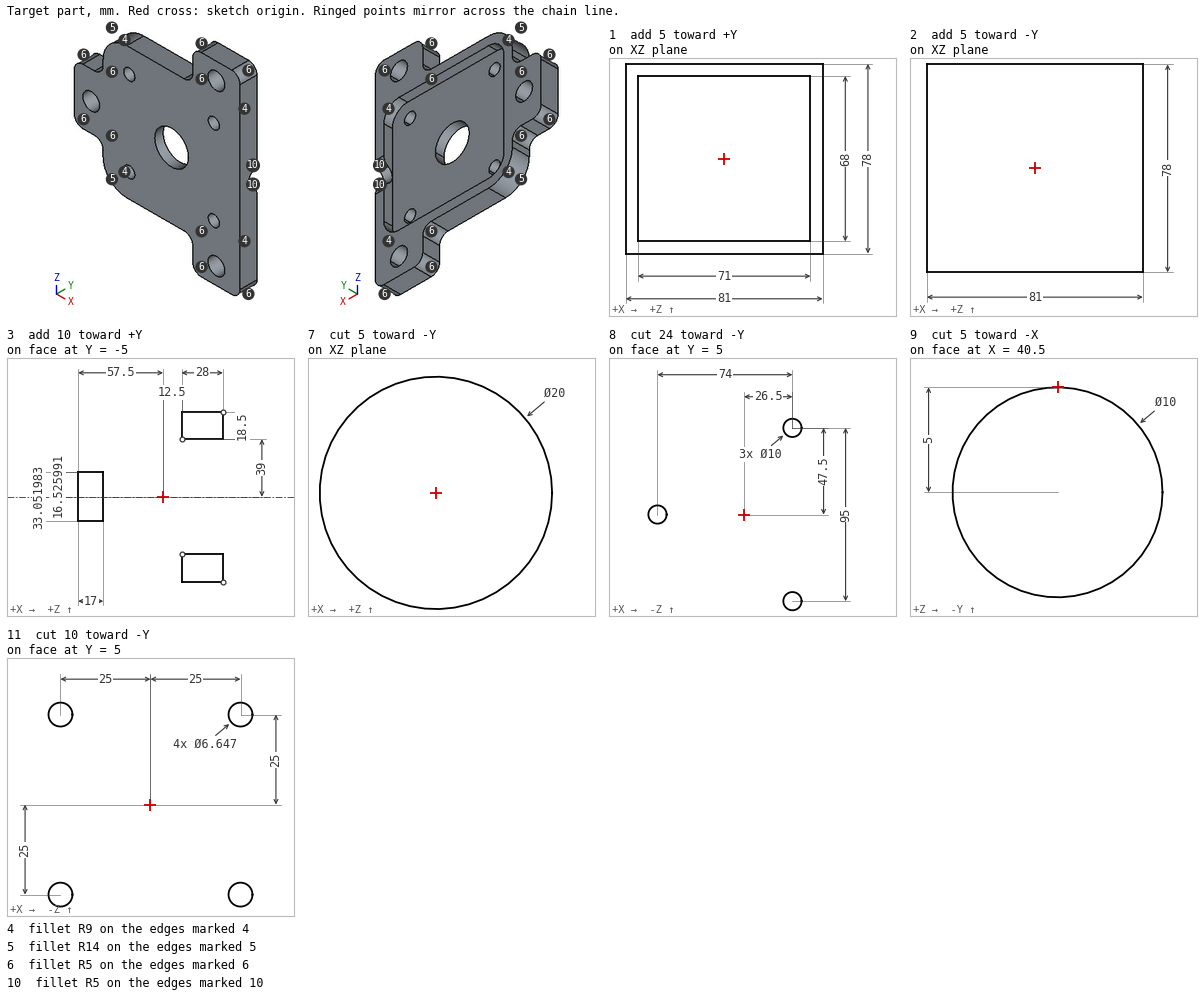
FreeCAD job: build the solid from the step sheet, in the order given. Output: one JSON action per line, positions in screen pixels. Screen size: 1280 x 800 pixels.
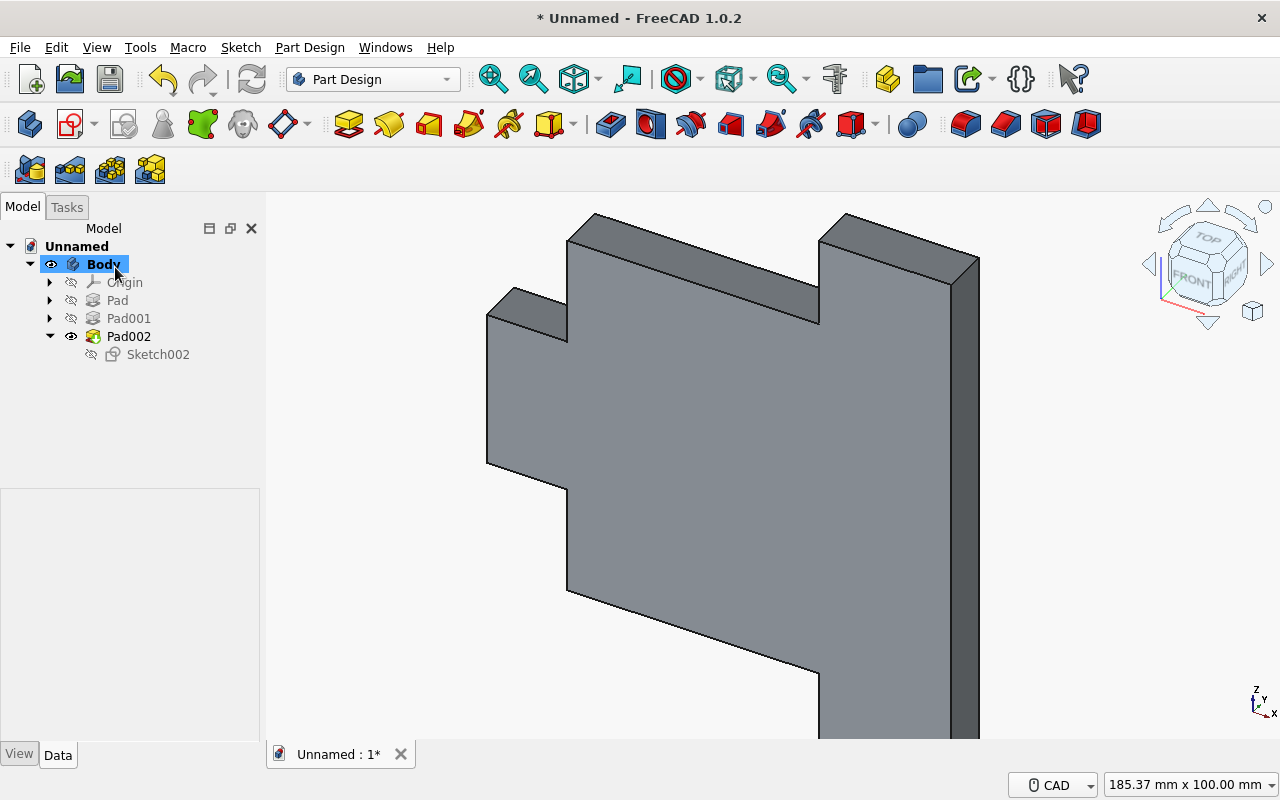
{"action": "key", "text": "v f"}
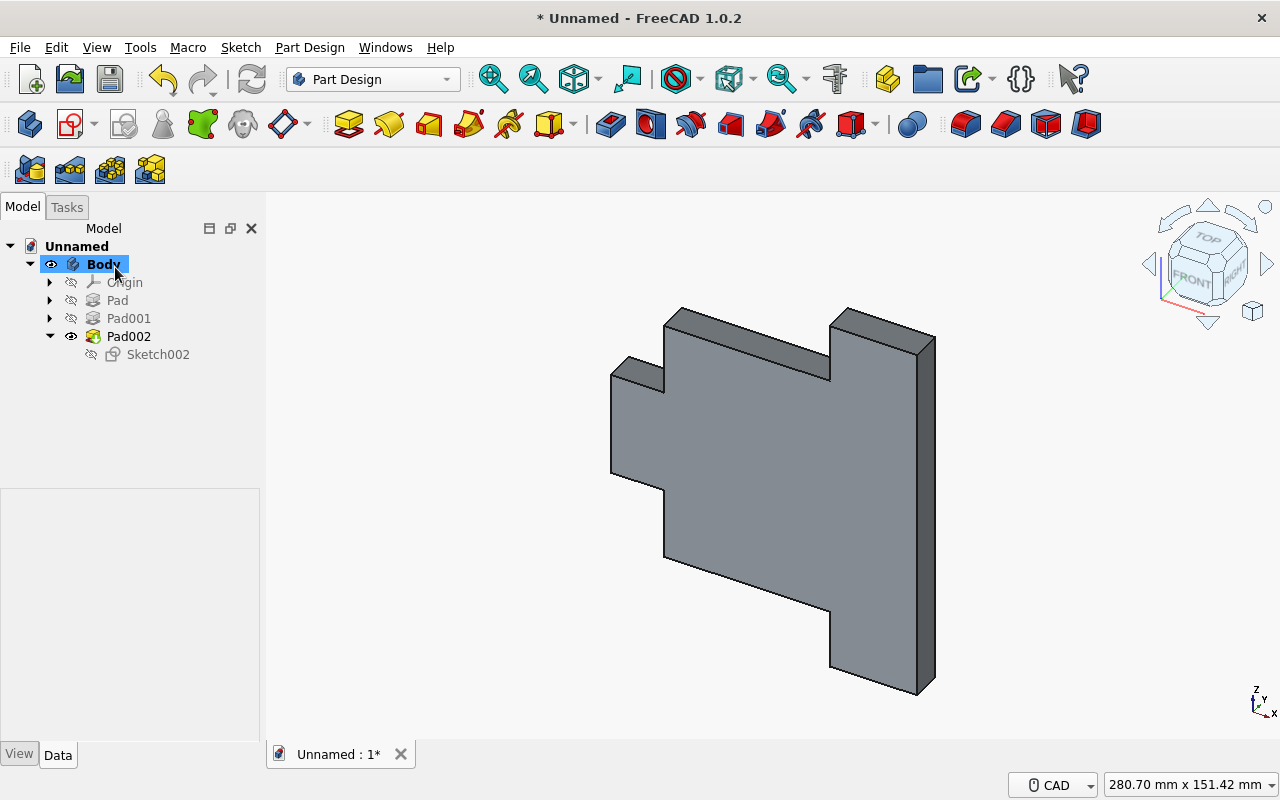
{"action": "scroll", "coordinate": [915, 405], "scroll_direction": "up", "scroll_amount": 4}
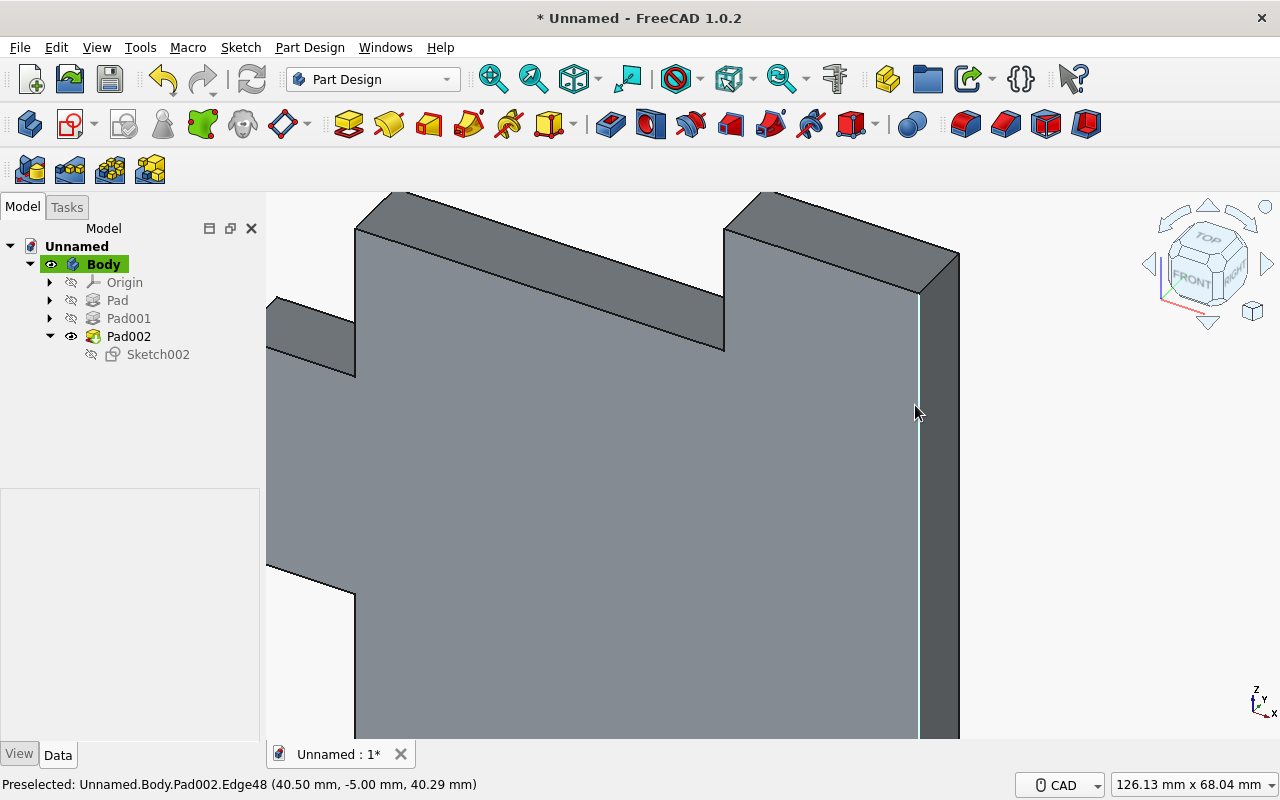
{"action": "key", "text": "v f"}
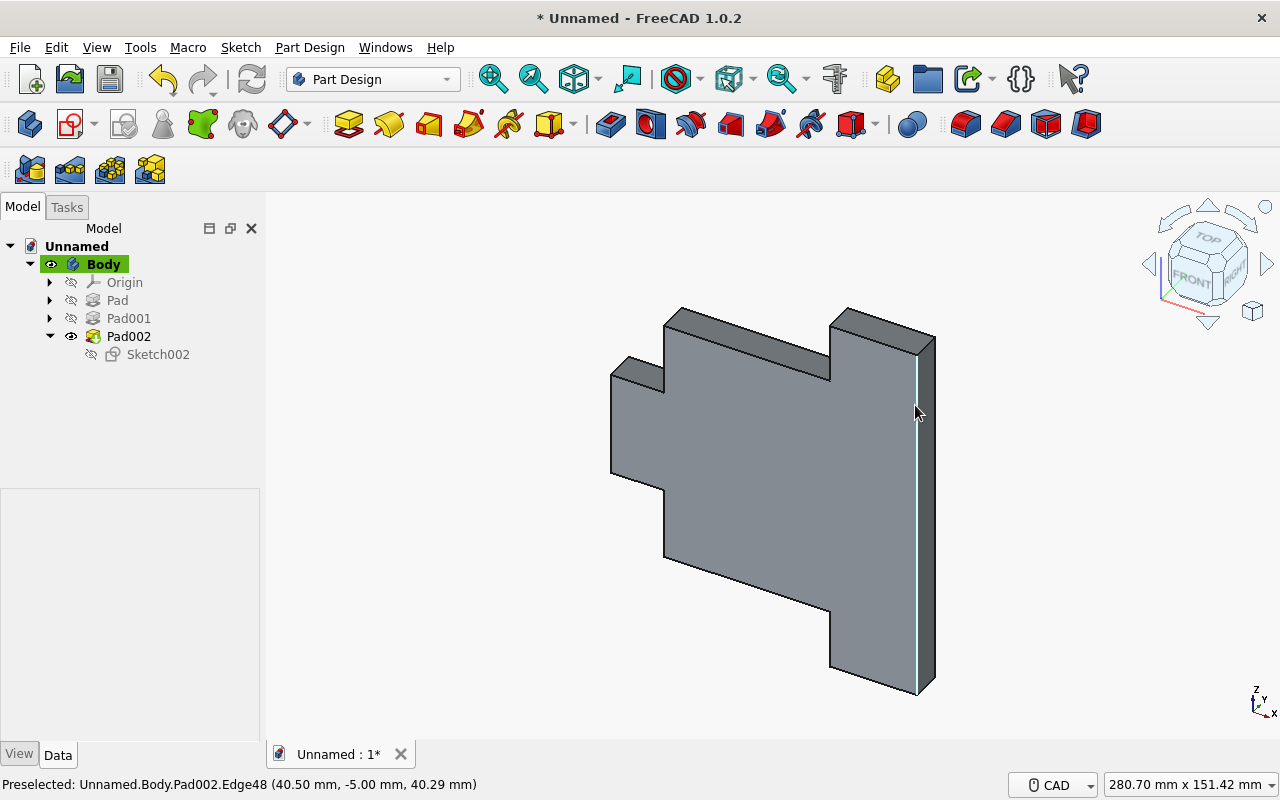
{"action": "key", "text": "0"}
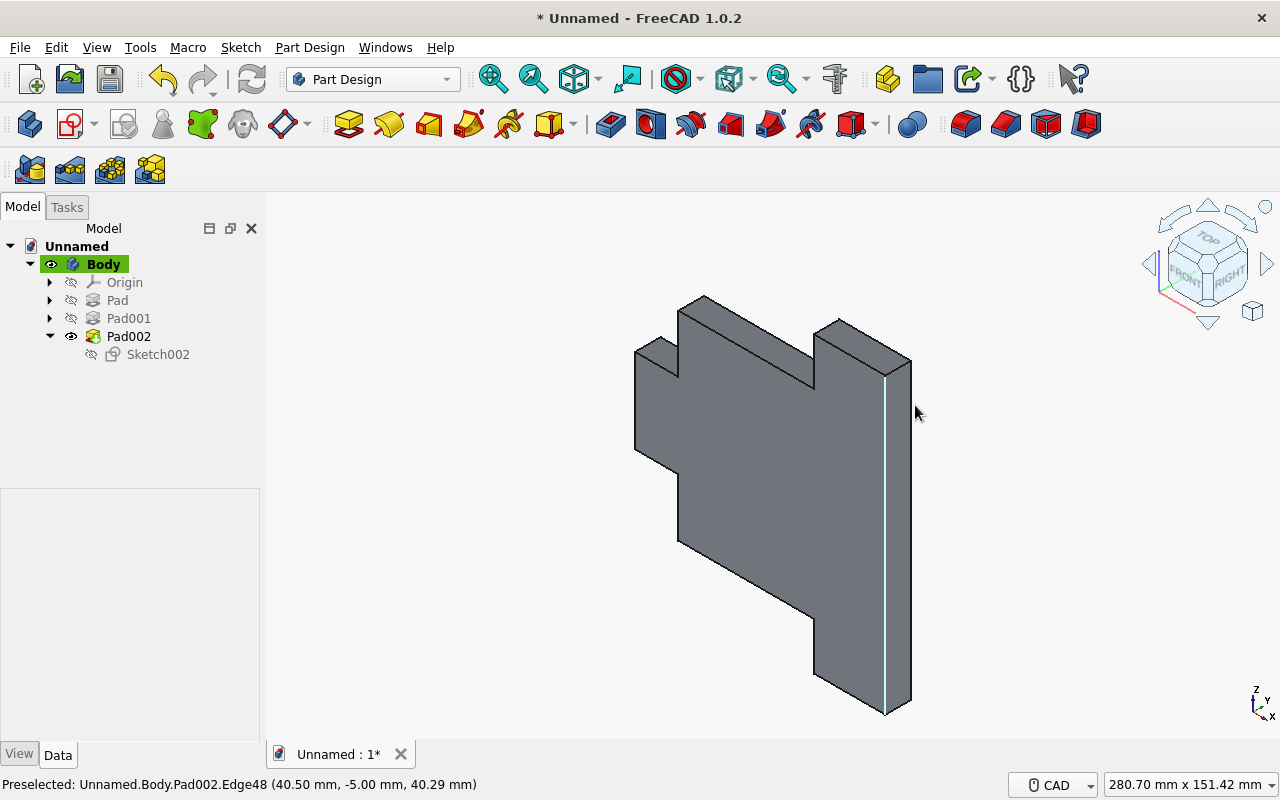
{"action": "scroll", "coordinate": [892, 425], "scroll_direction": "up", "scroll_amount": 4}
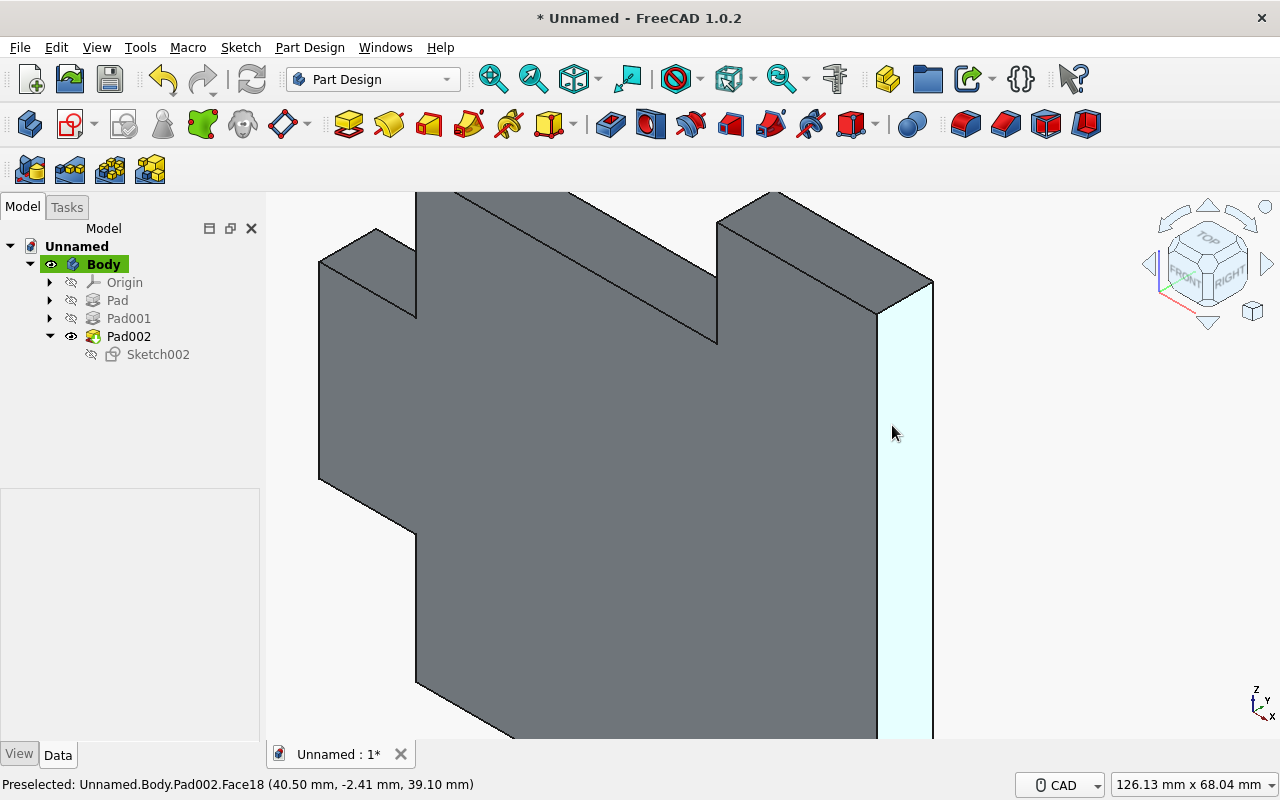
{"action": "key", "text": "v f"}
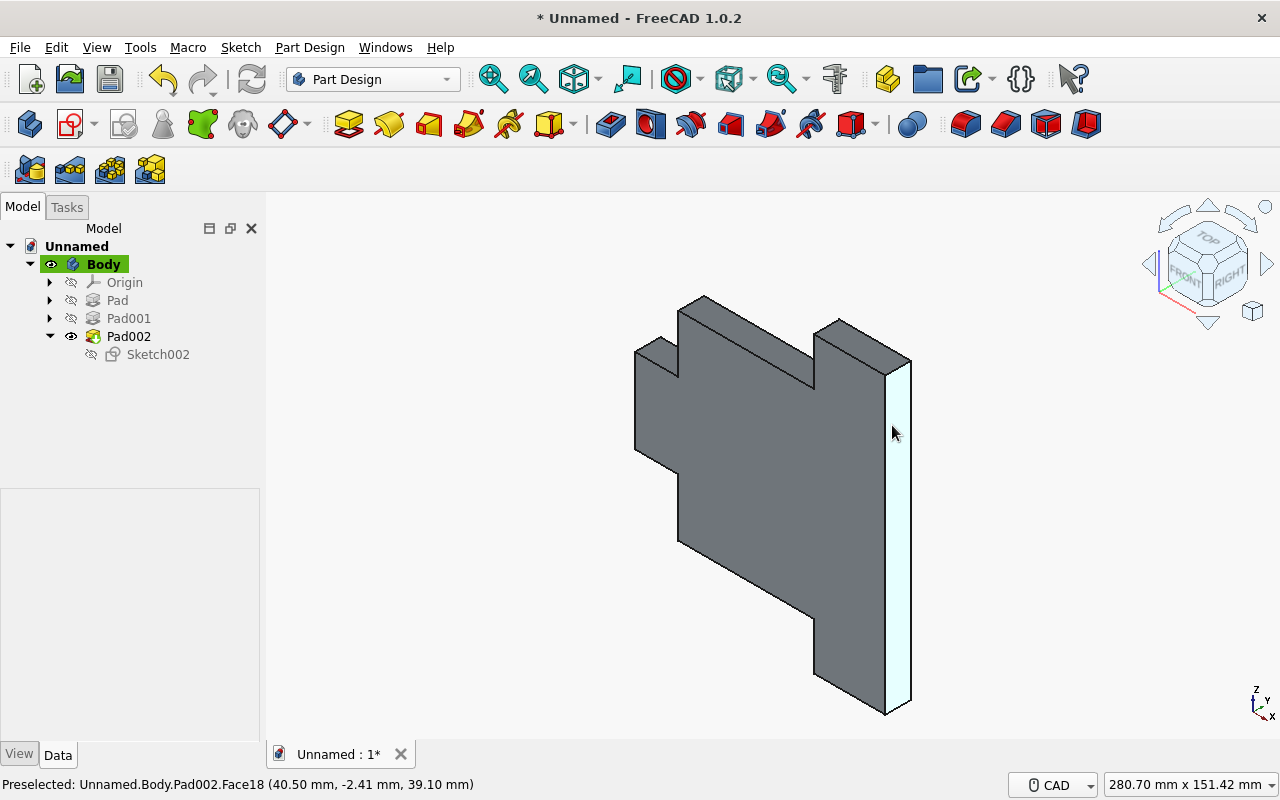
{"action": "key", "text": "2"}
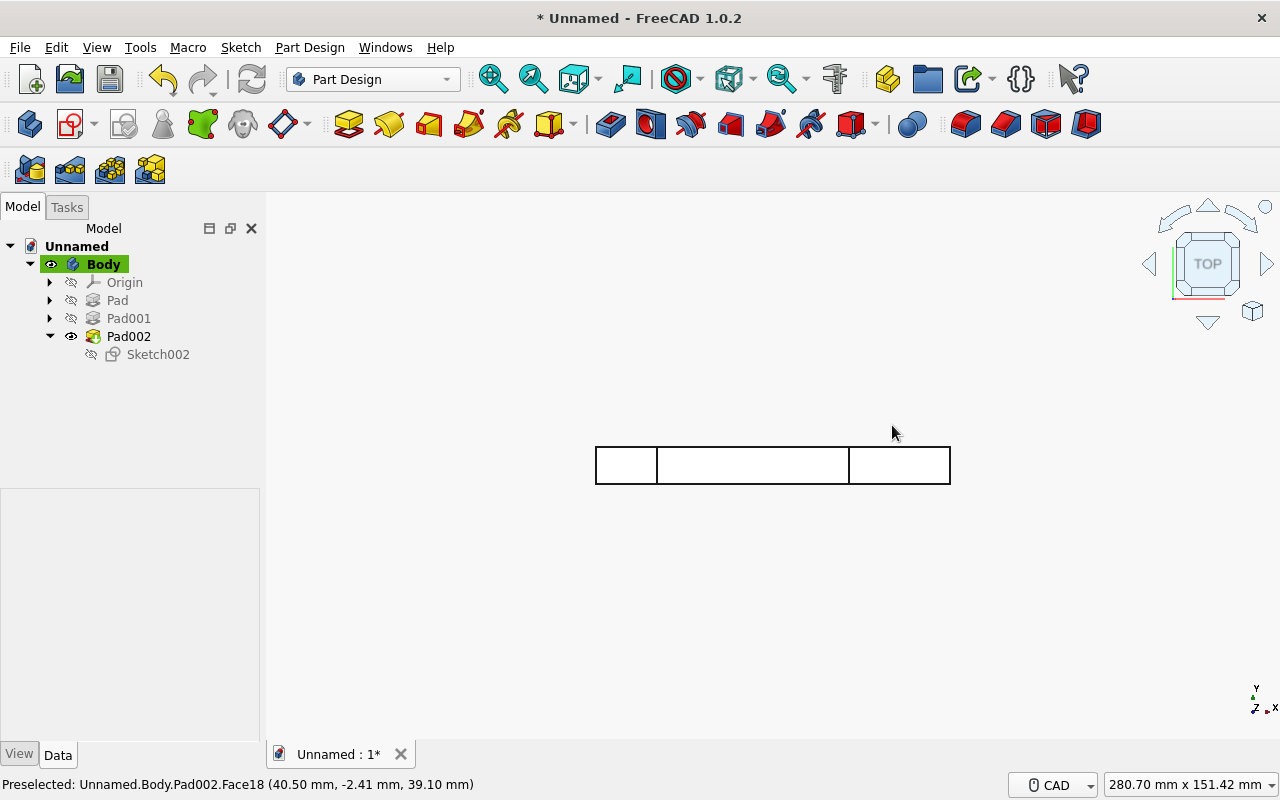
{"action": "left_click", "coordinate": [494, 80]}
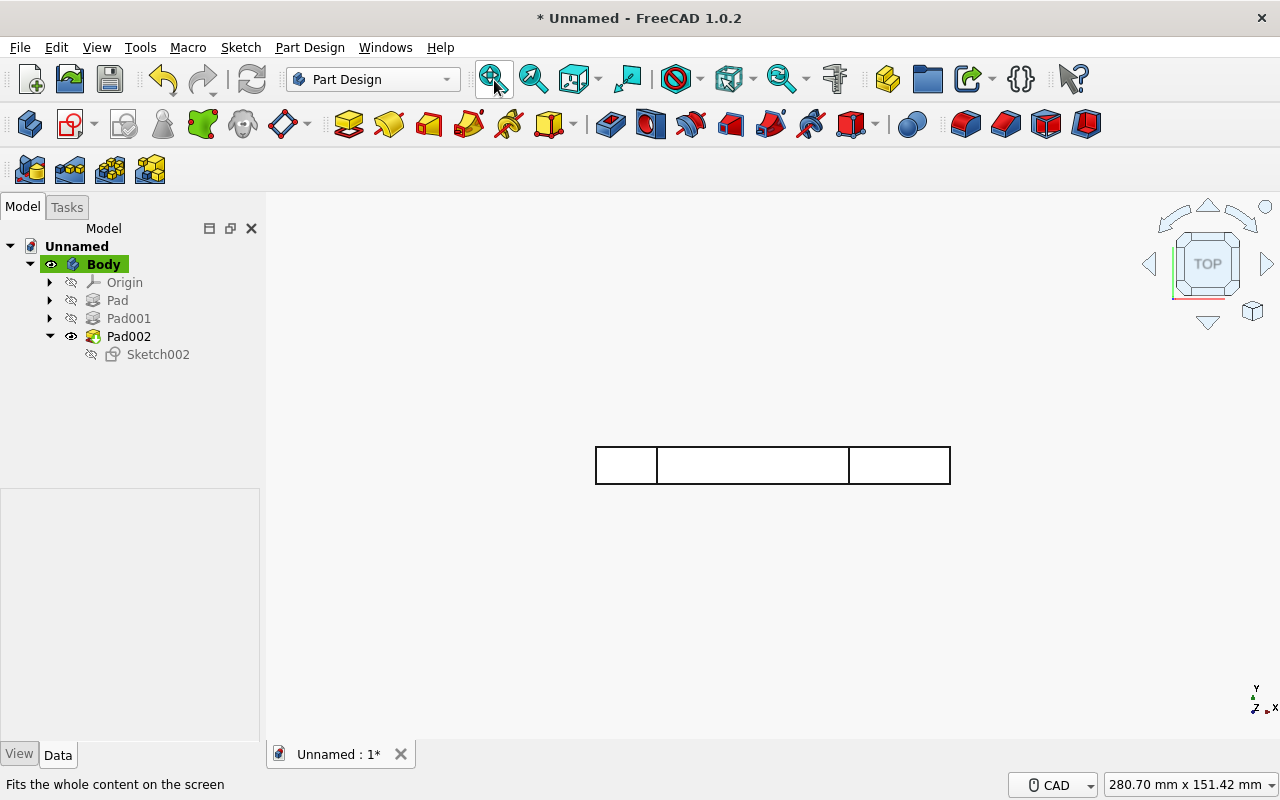
{"action": "scroll", "coordinate": [932, 455], "scroll_direction": "up", "scroll_amount": 4}